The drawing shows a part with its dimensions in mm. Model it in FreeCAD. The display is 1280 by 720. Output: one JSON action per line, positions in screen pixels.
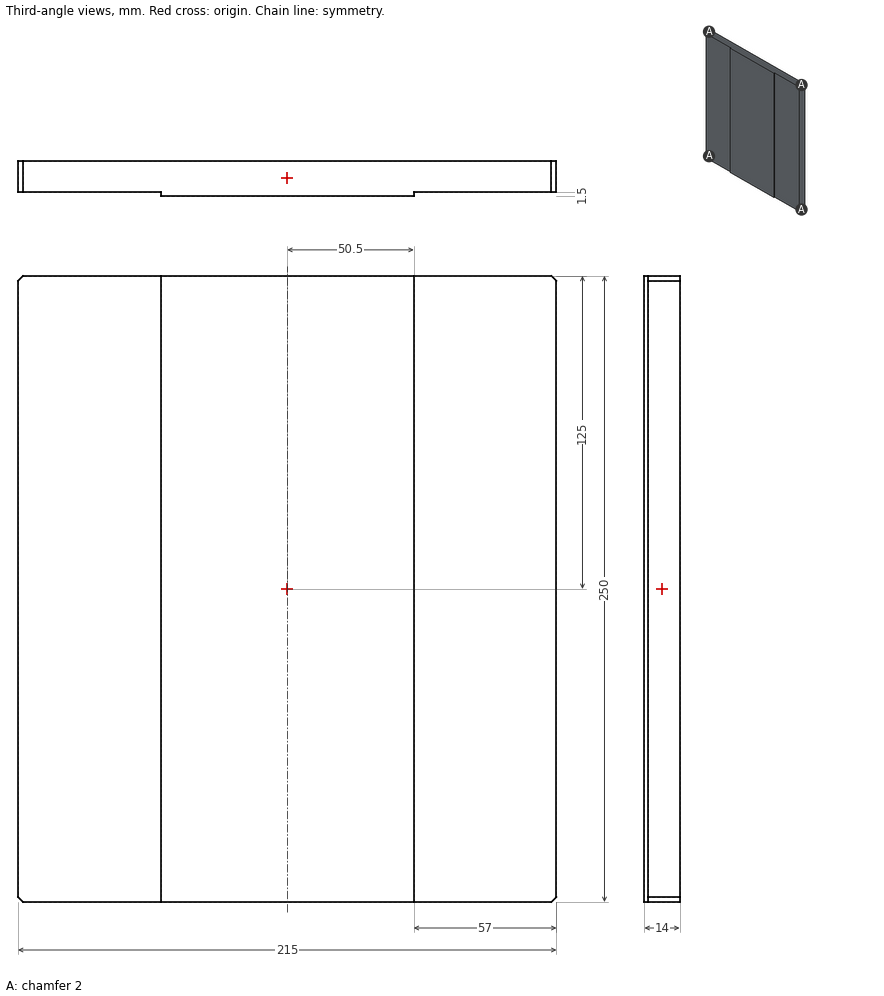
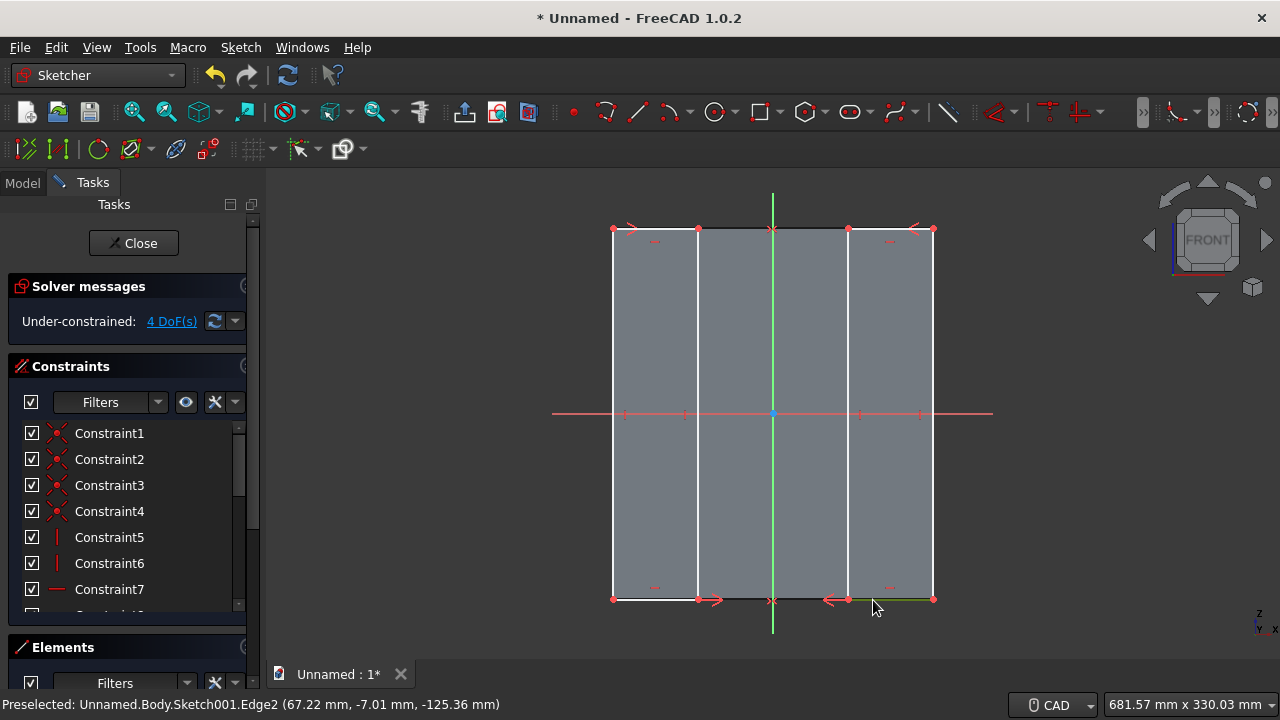
{"action": "key", "text": "l"}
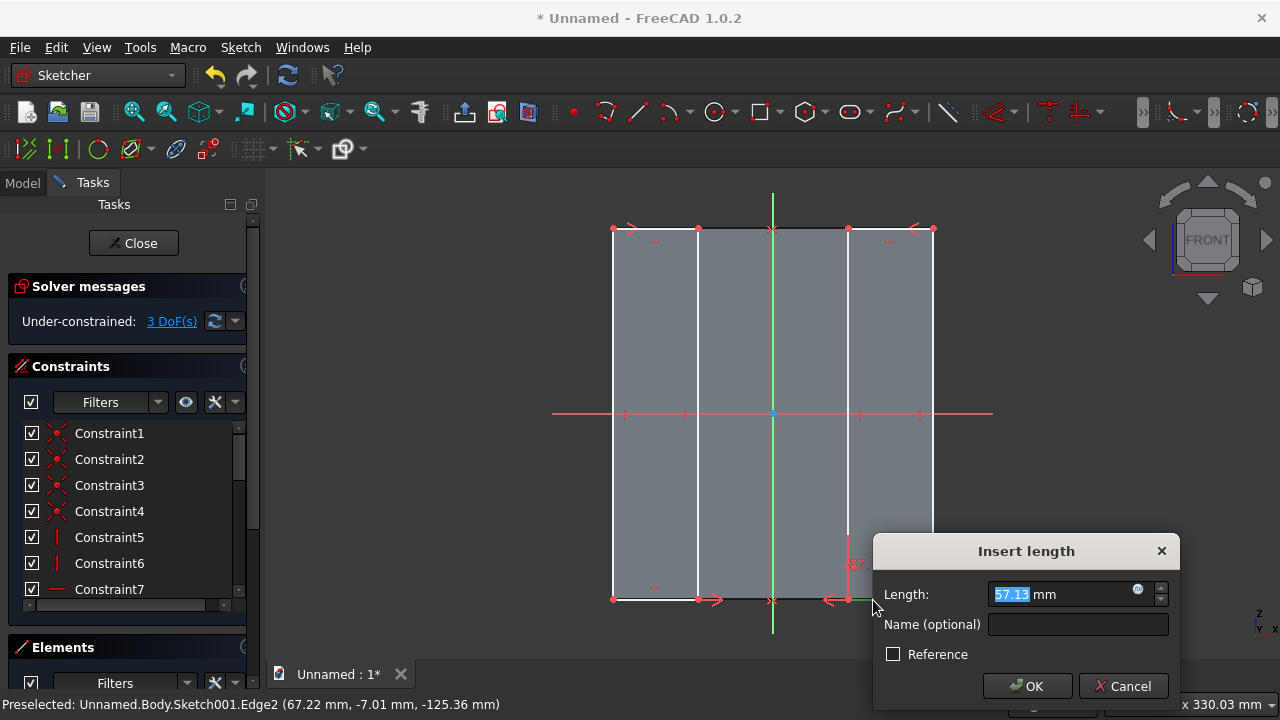
{"action": "type", "text": "57"}
{"action": "key", "text": "Return"}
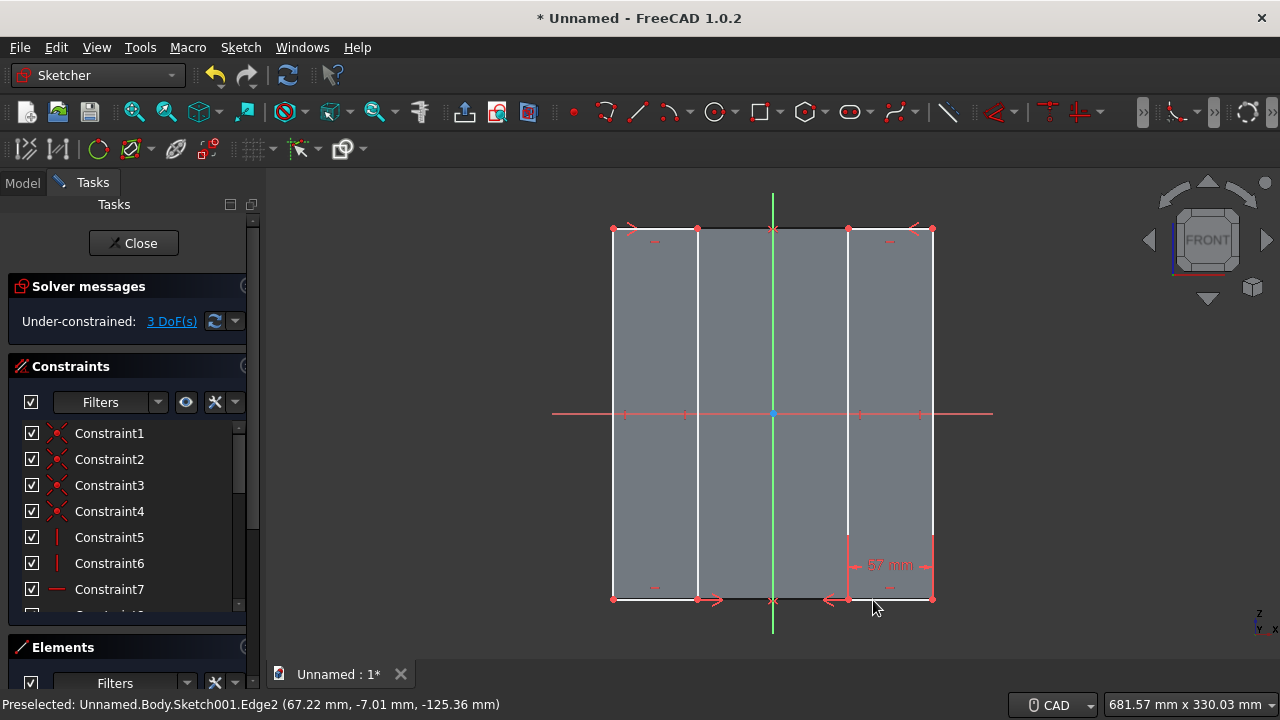
{"action": "left_click", "coordinate": [848, 340]}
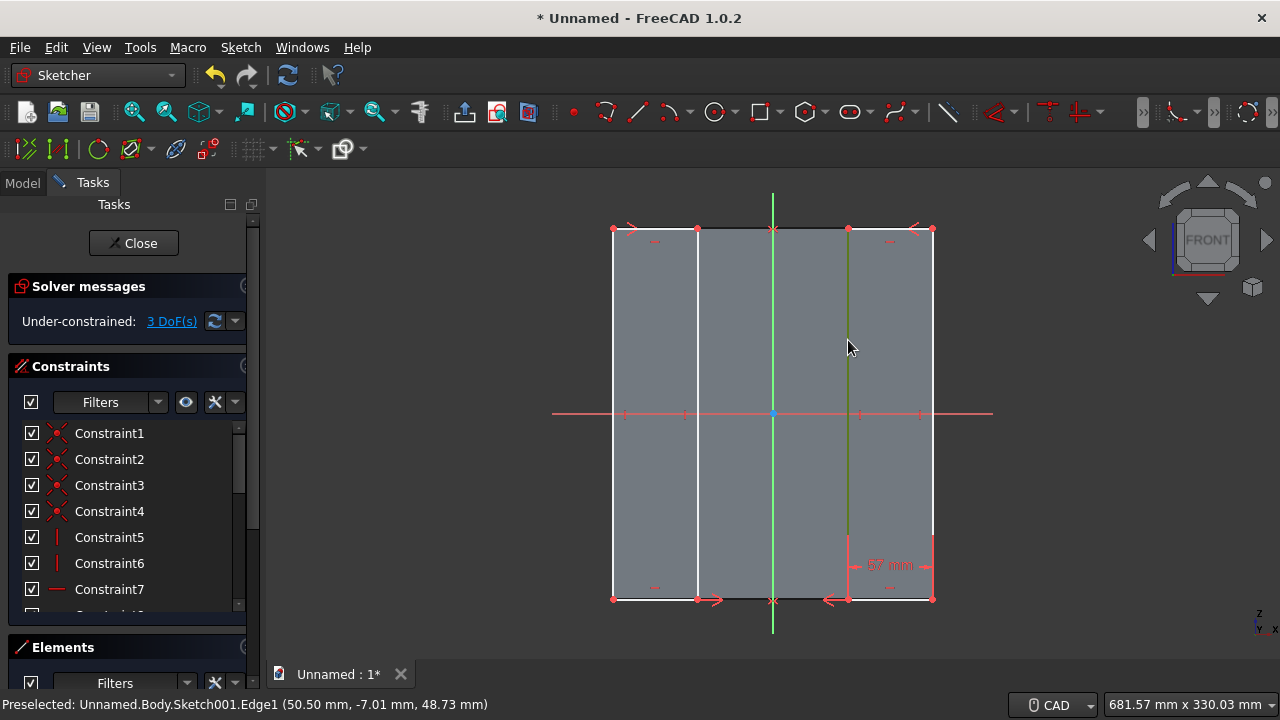
{"action": "key", "text": "i"}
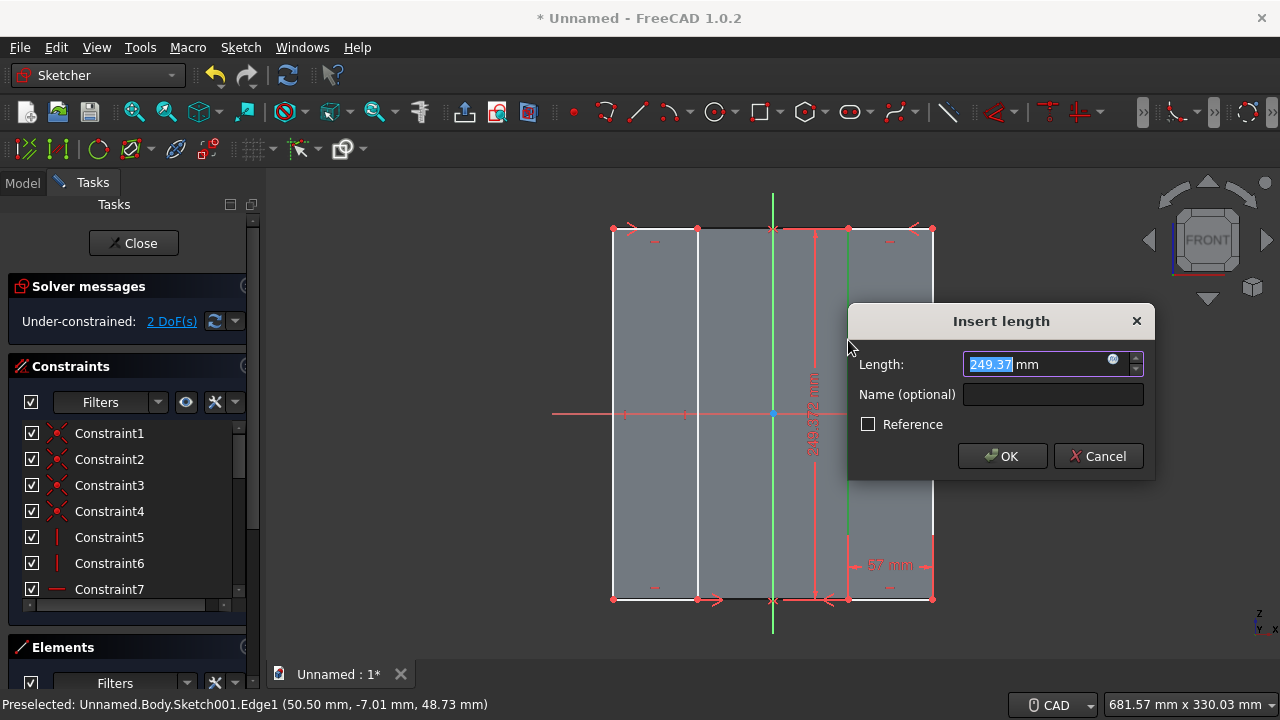
{"action": "type", "text": "250"}
{"action": "key", "text": "Return"}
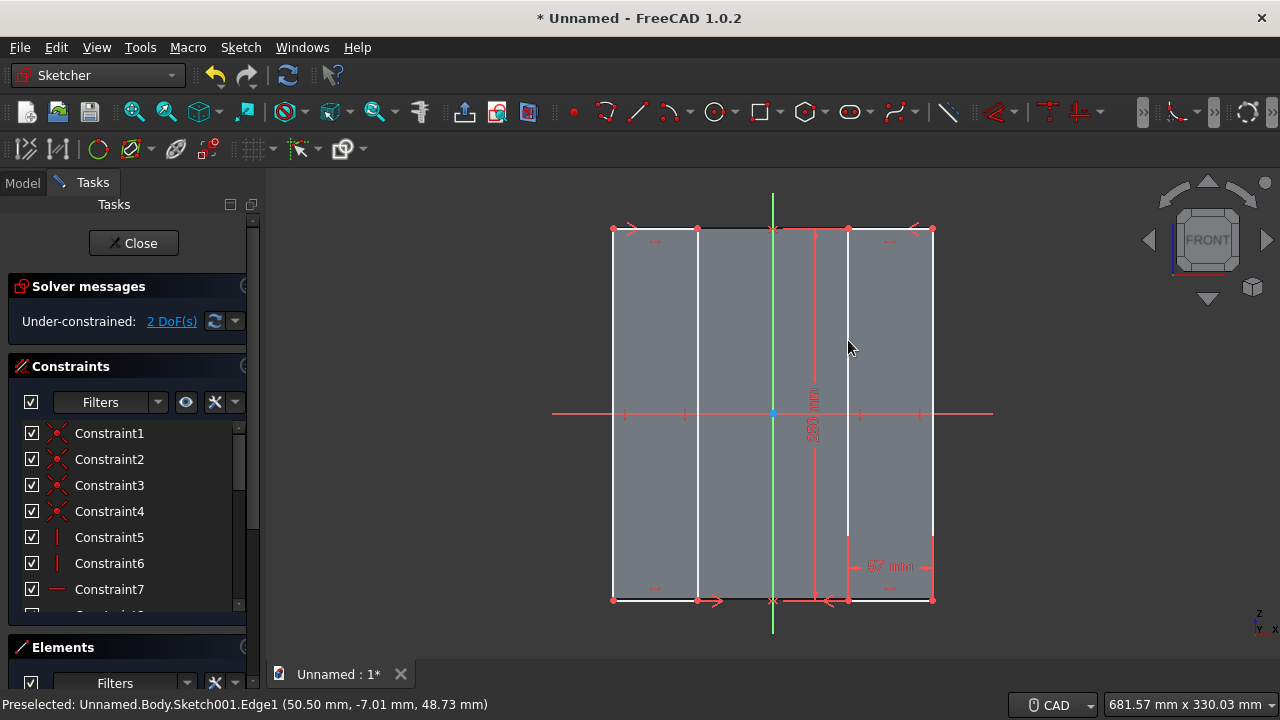
{"action": "left_click", "coordinate": [848, 229]}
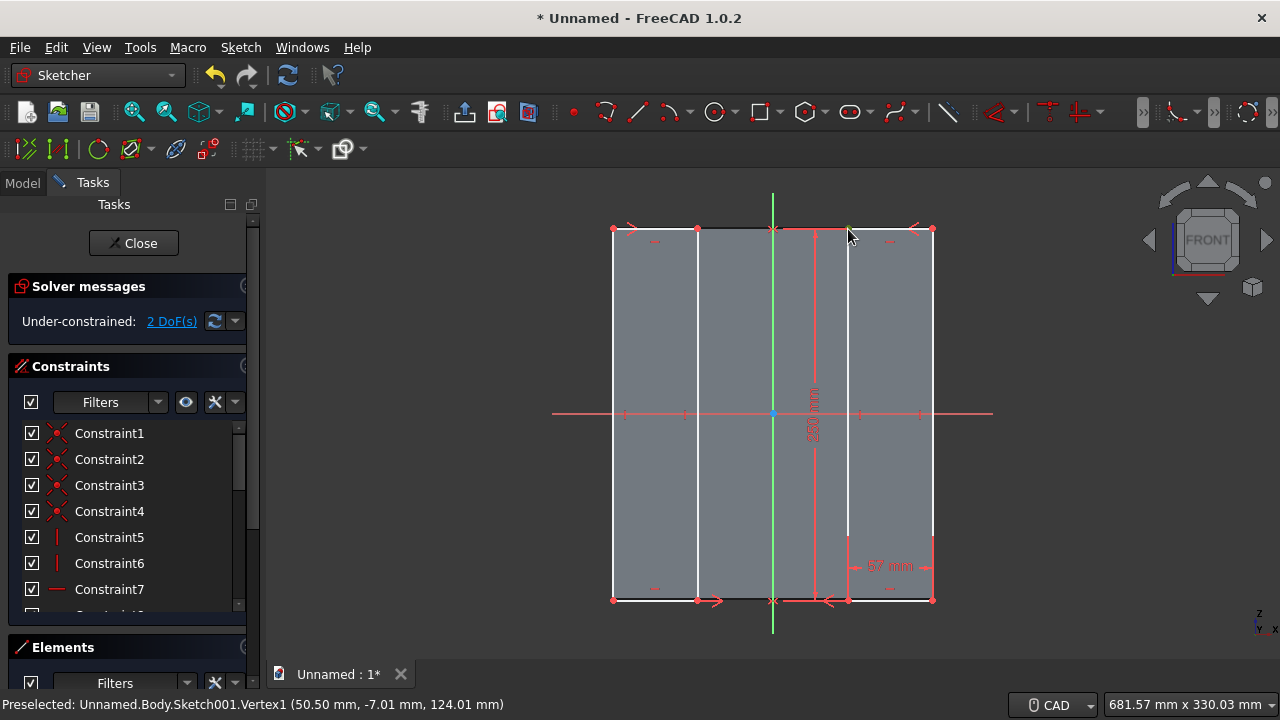
{"action": "key", "text": "i"}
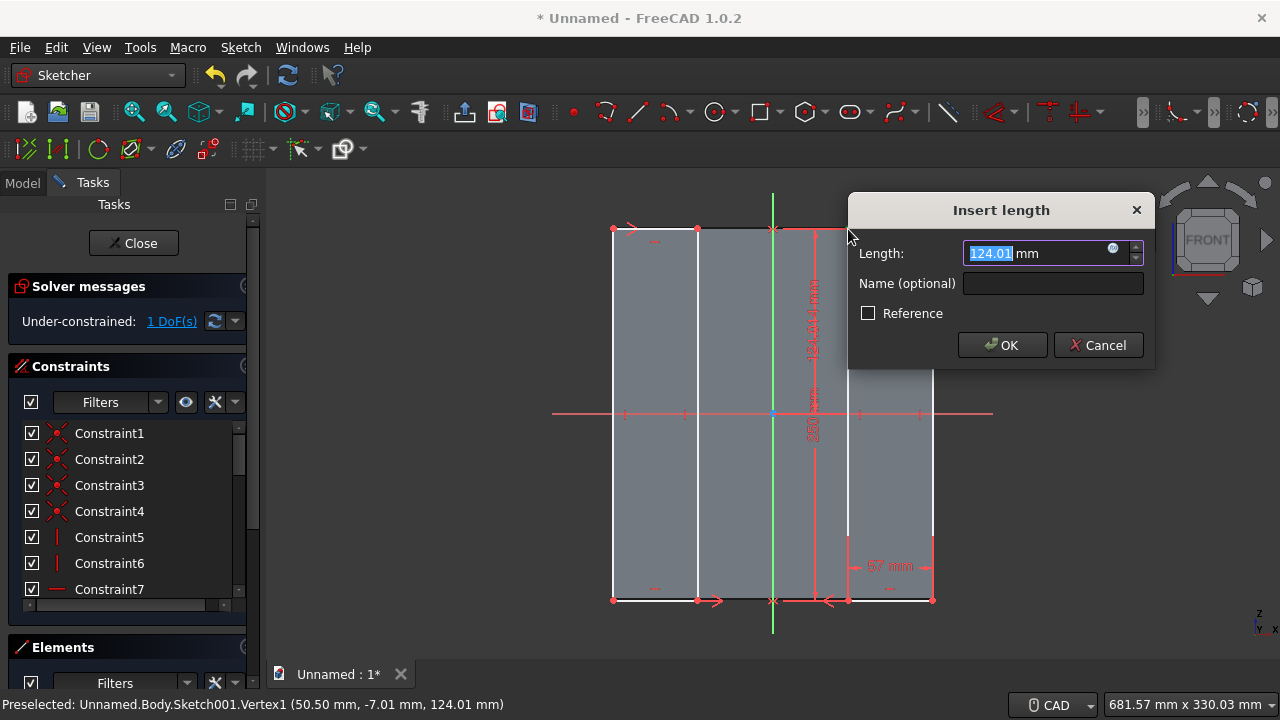
{"action": "type", "text": "125"}
{"action": "key", "text": "Return"}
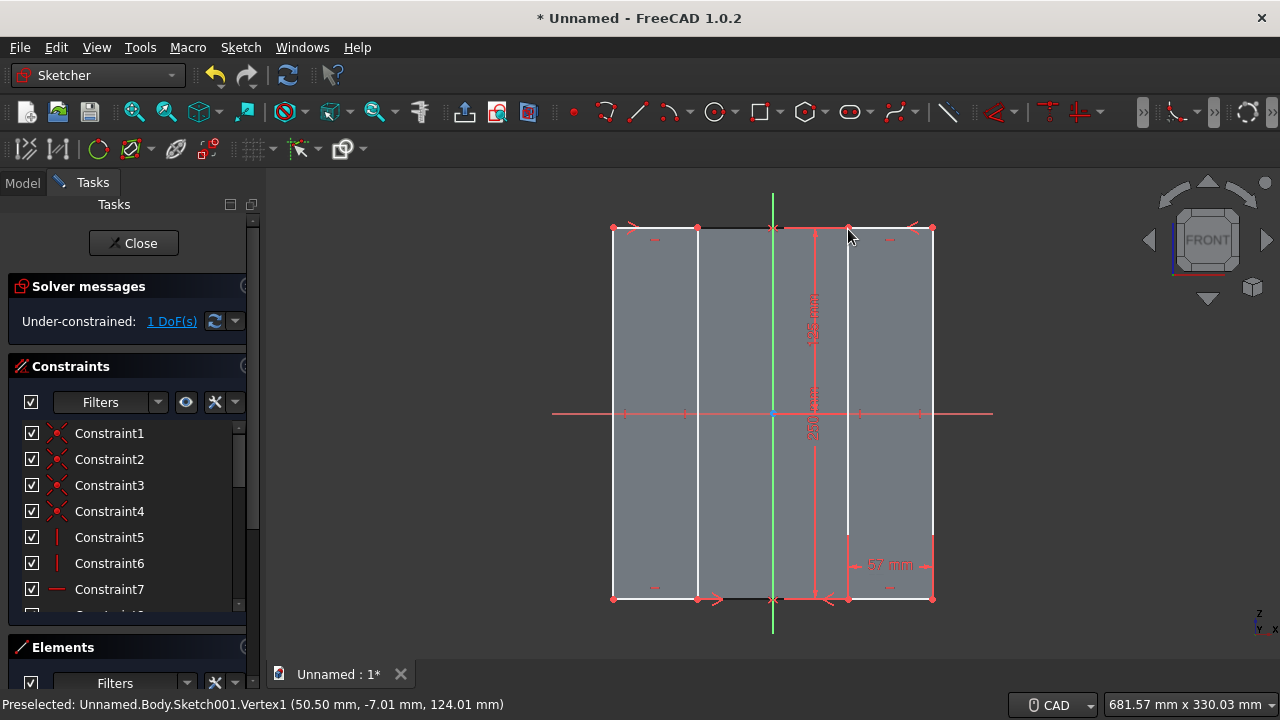
{"action": "left_click", "coordinate": [848, 228]}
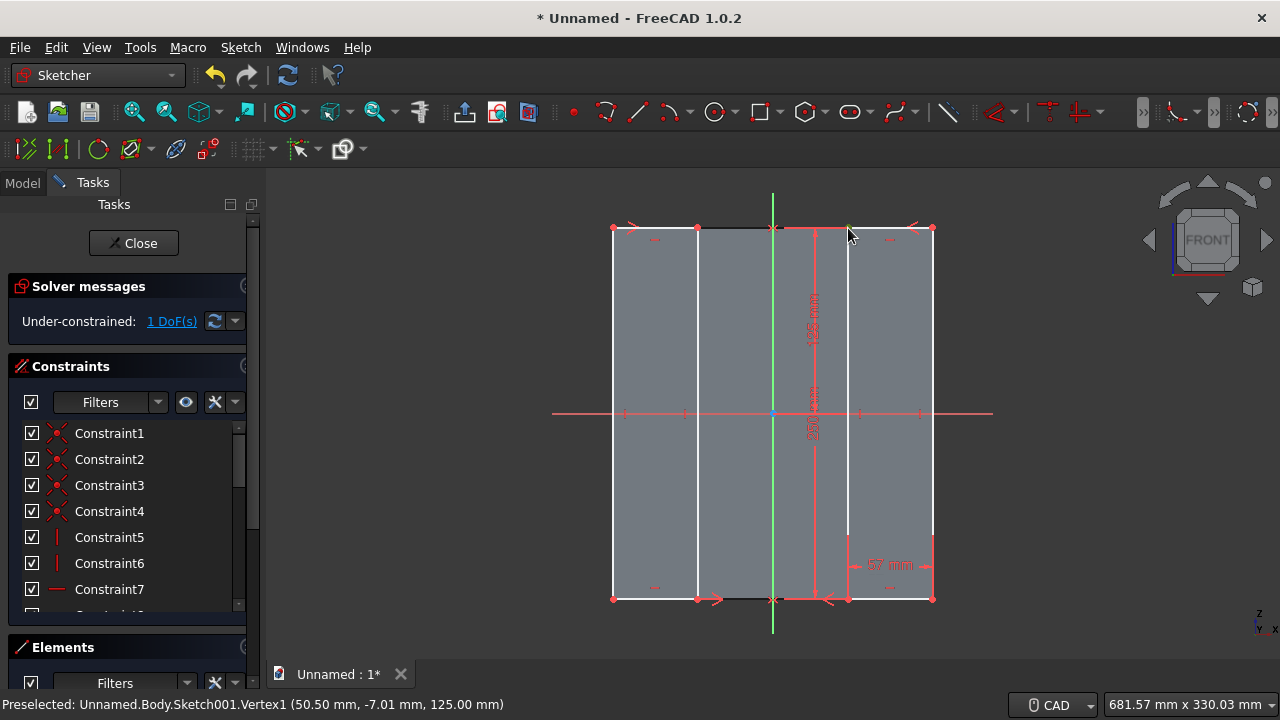
{"action": "key", "text": "l"}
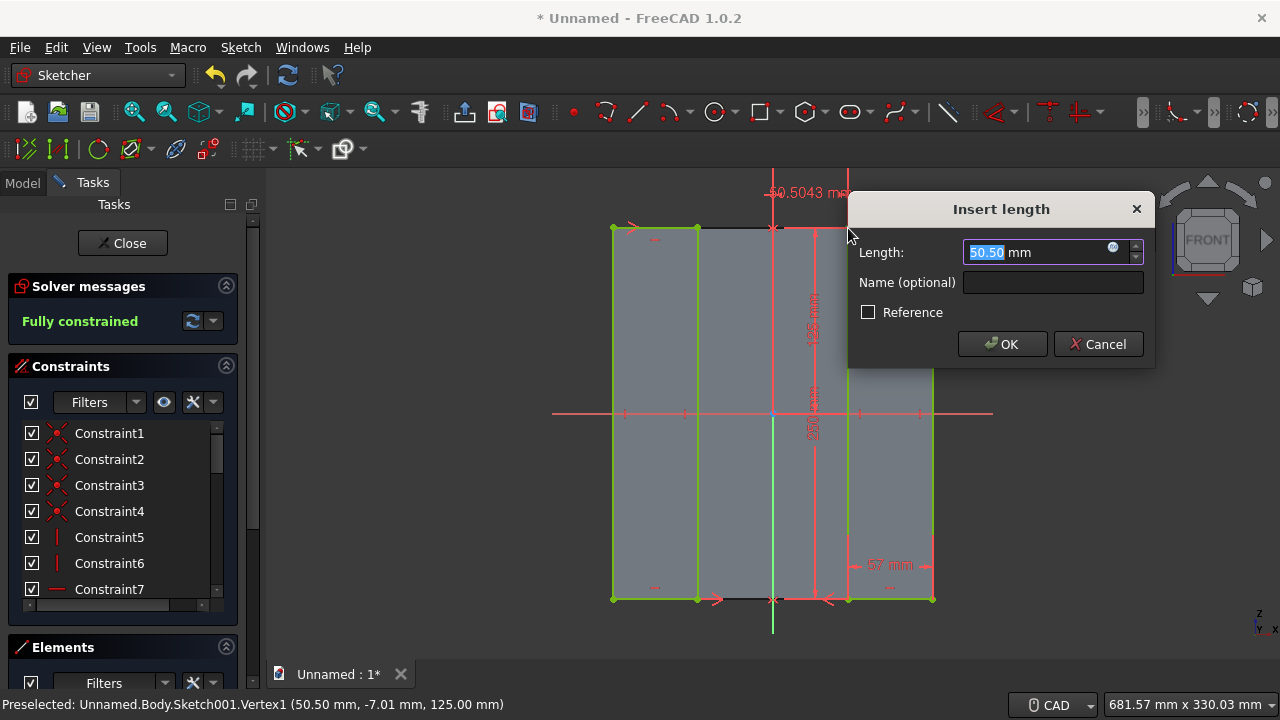
{"action": "type", "text": "50.5"}
{"action": "key", "text": "Return"}